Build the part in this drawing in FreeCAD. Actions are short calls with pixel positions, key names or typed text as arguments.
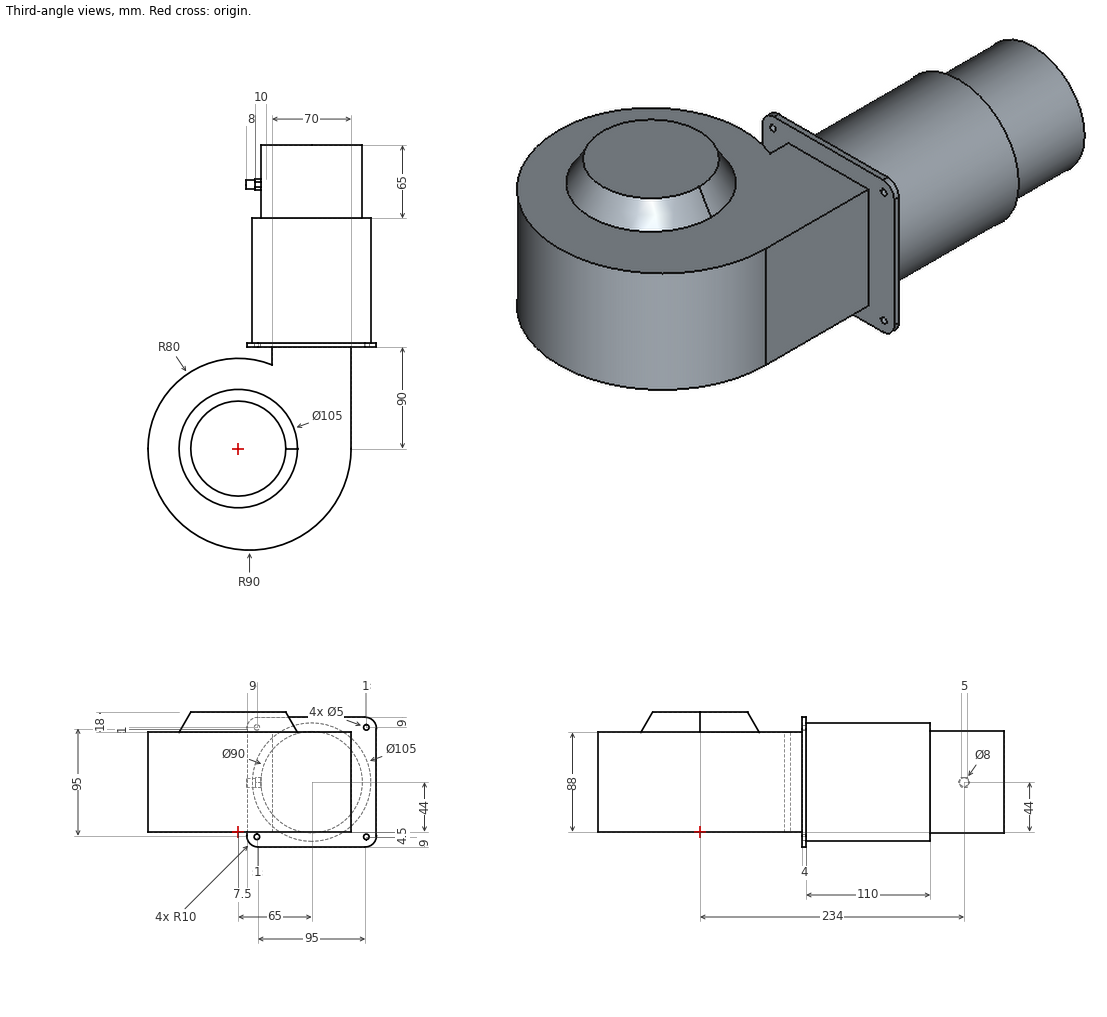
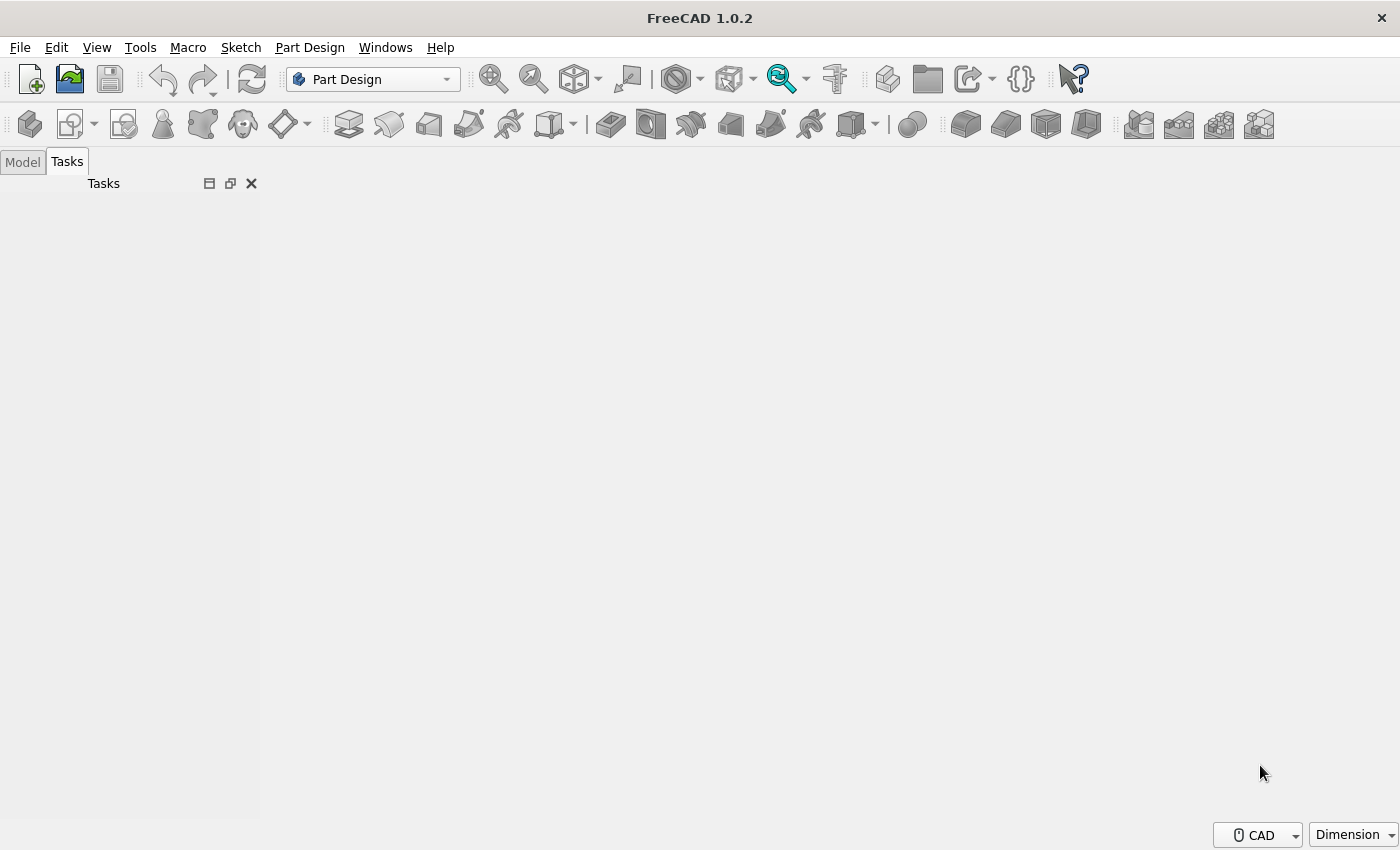
click(30, 80)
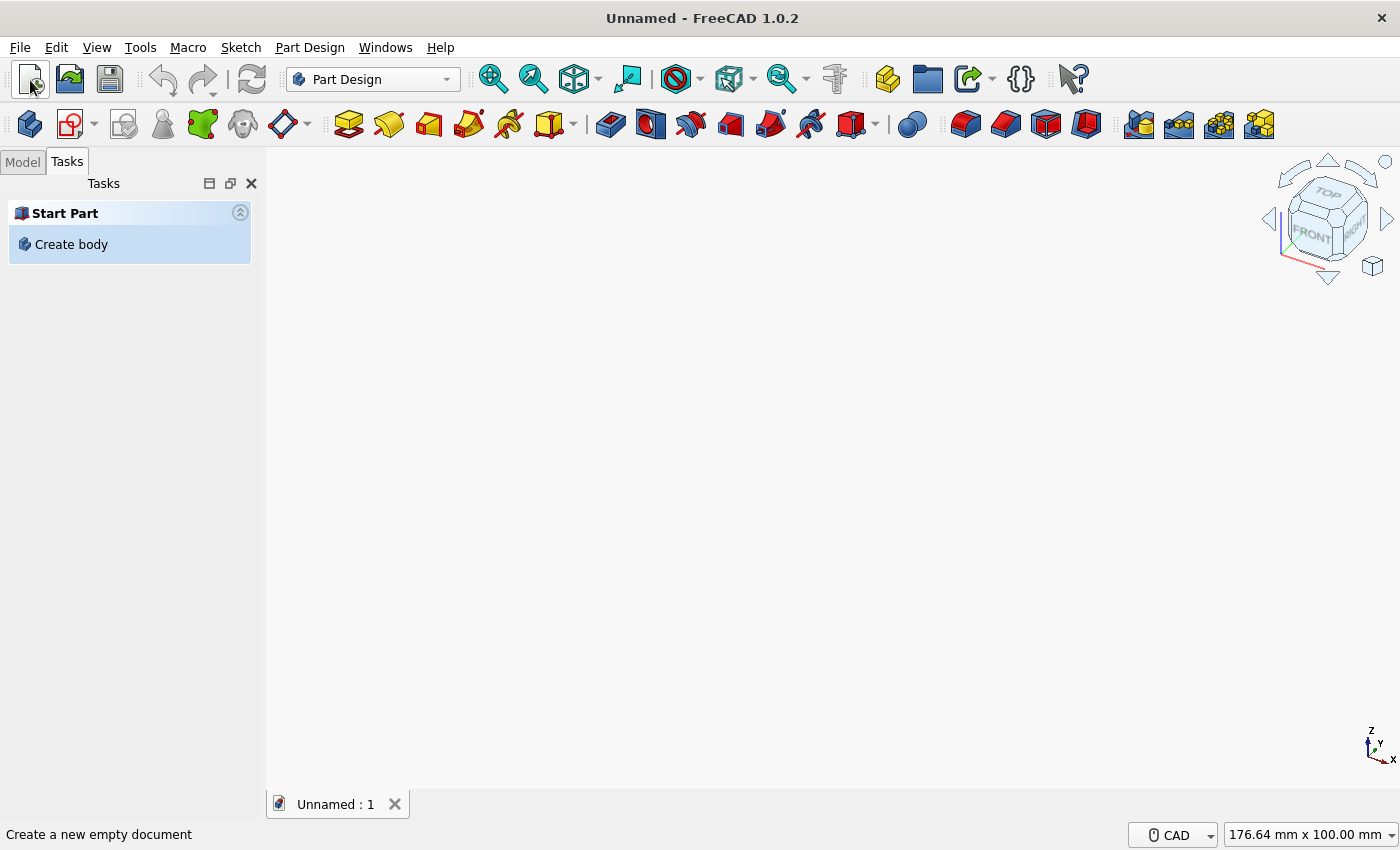
click(70, 124)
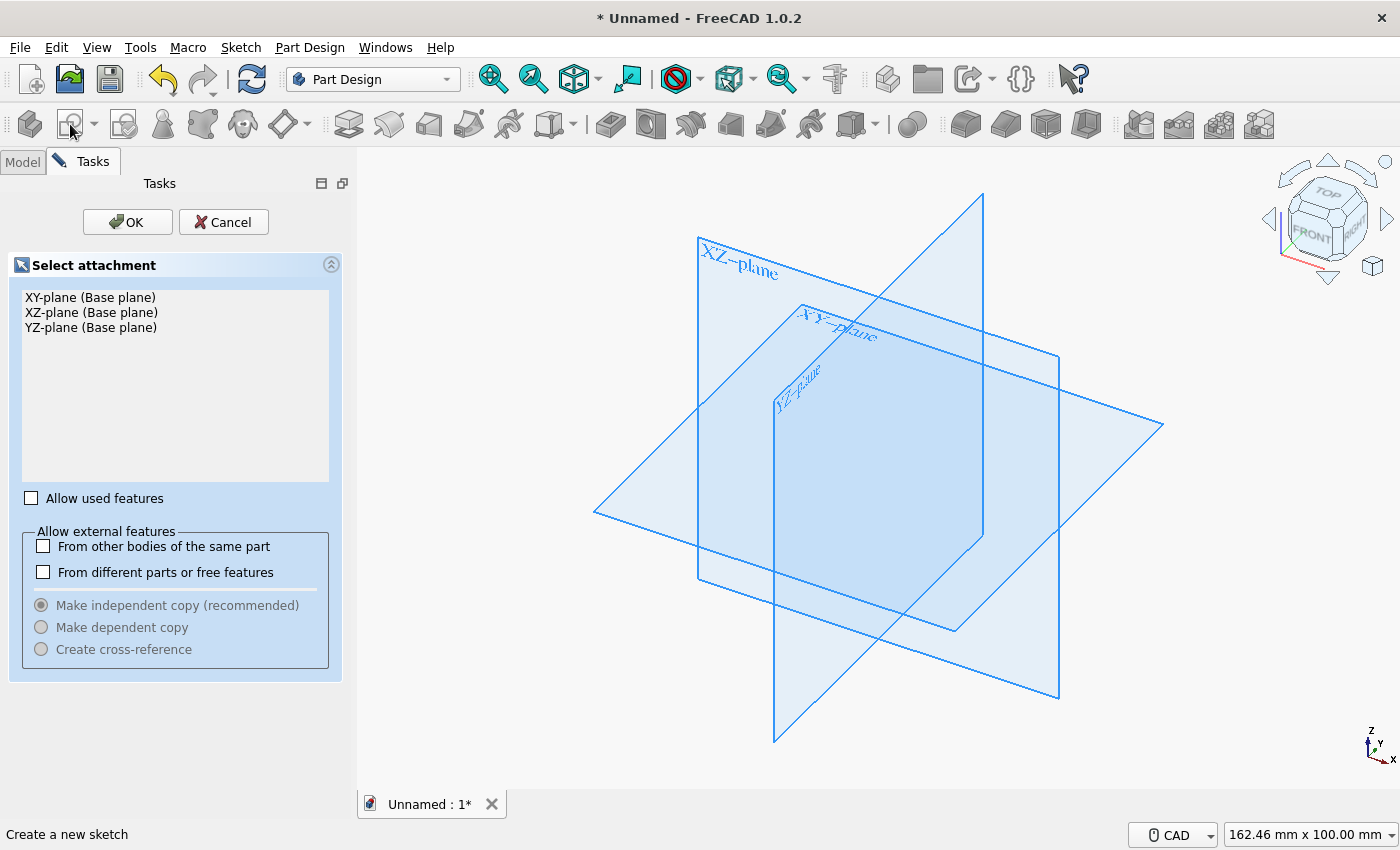
click(82, 298)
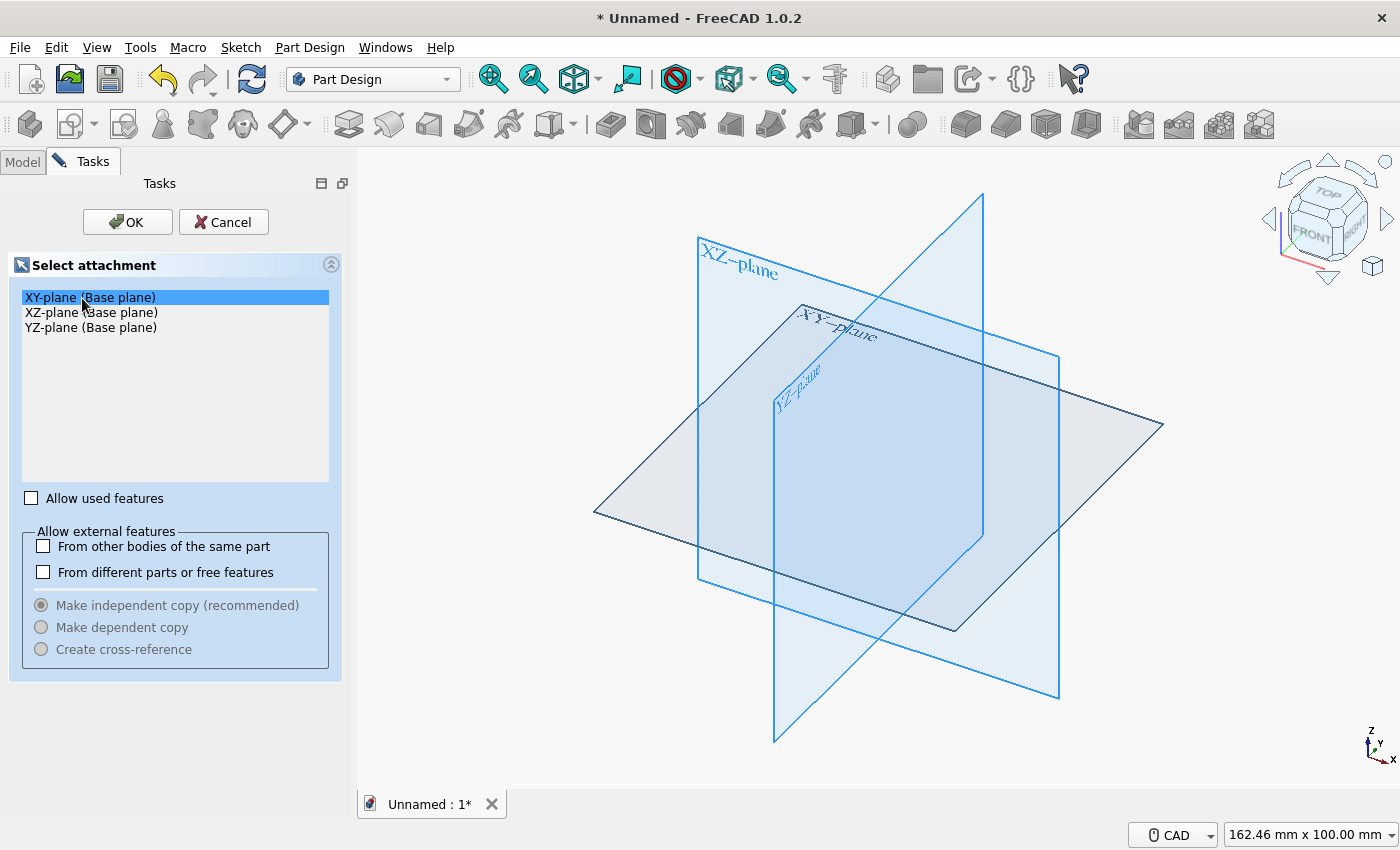
click(128, 222)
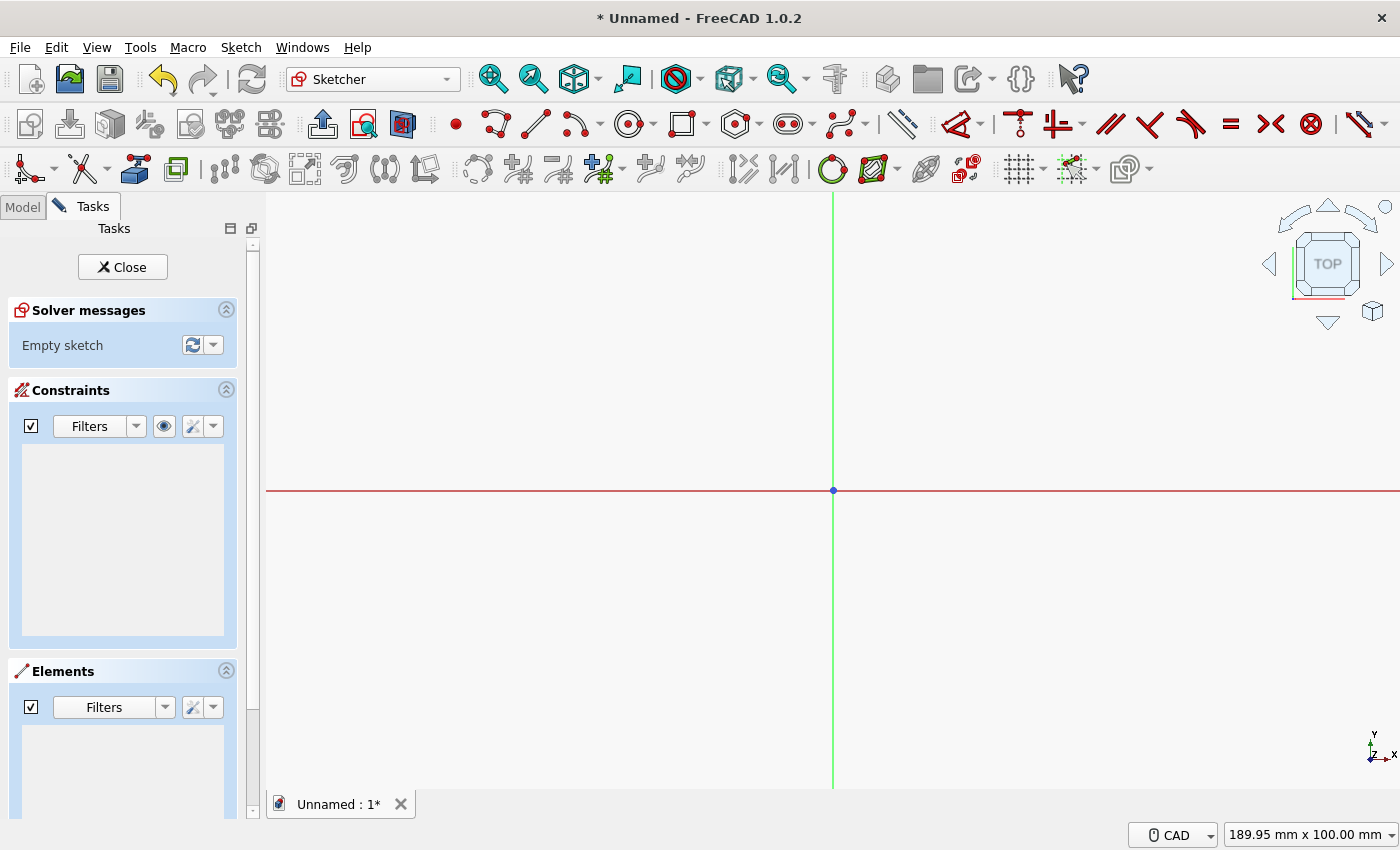
scroll(690, 490, down, 5)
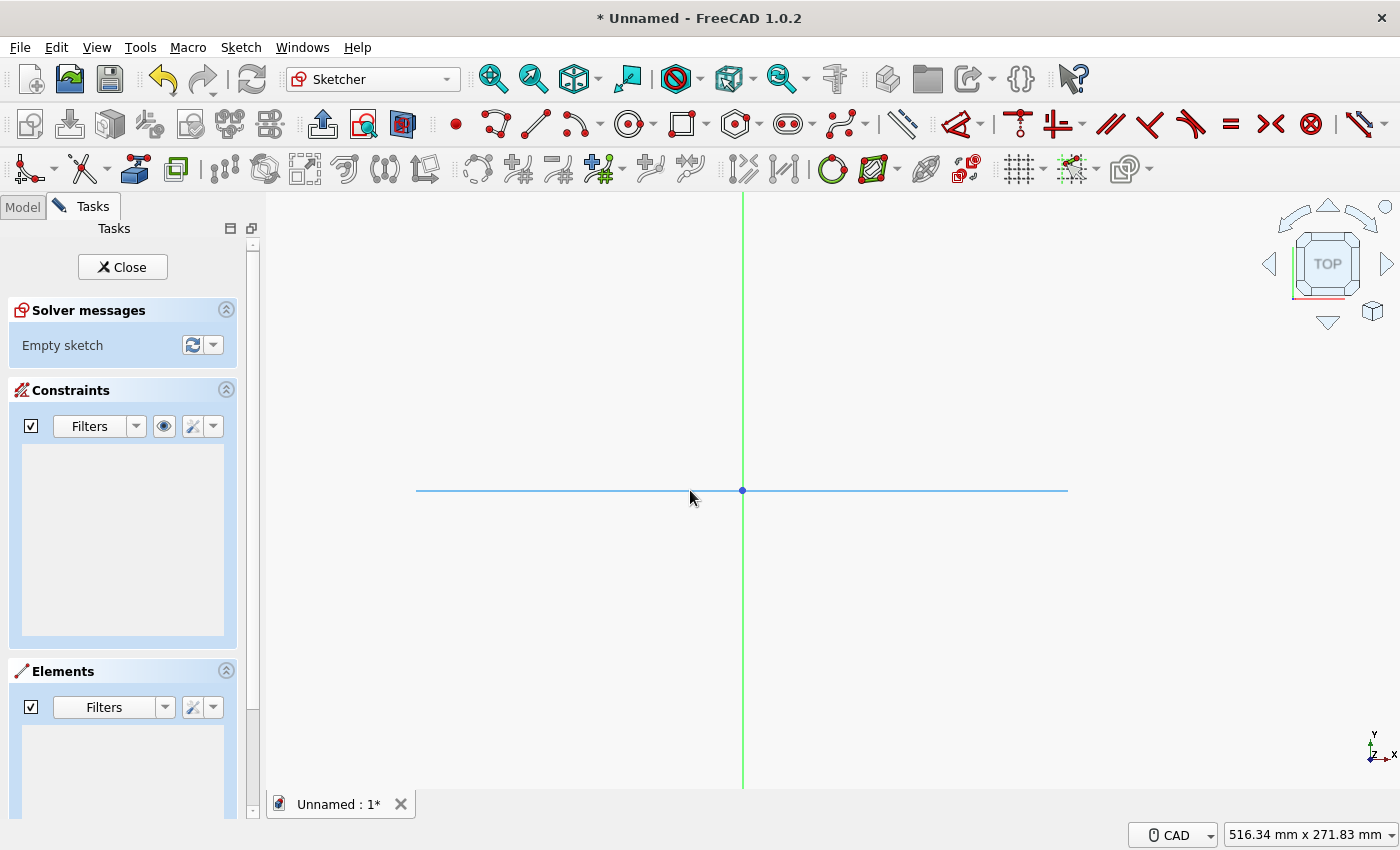
key(g)
key(m)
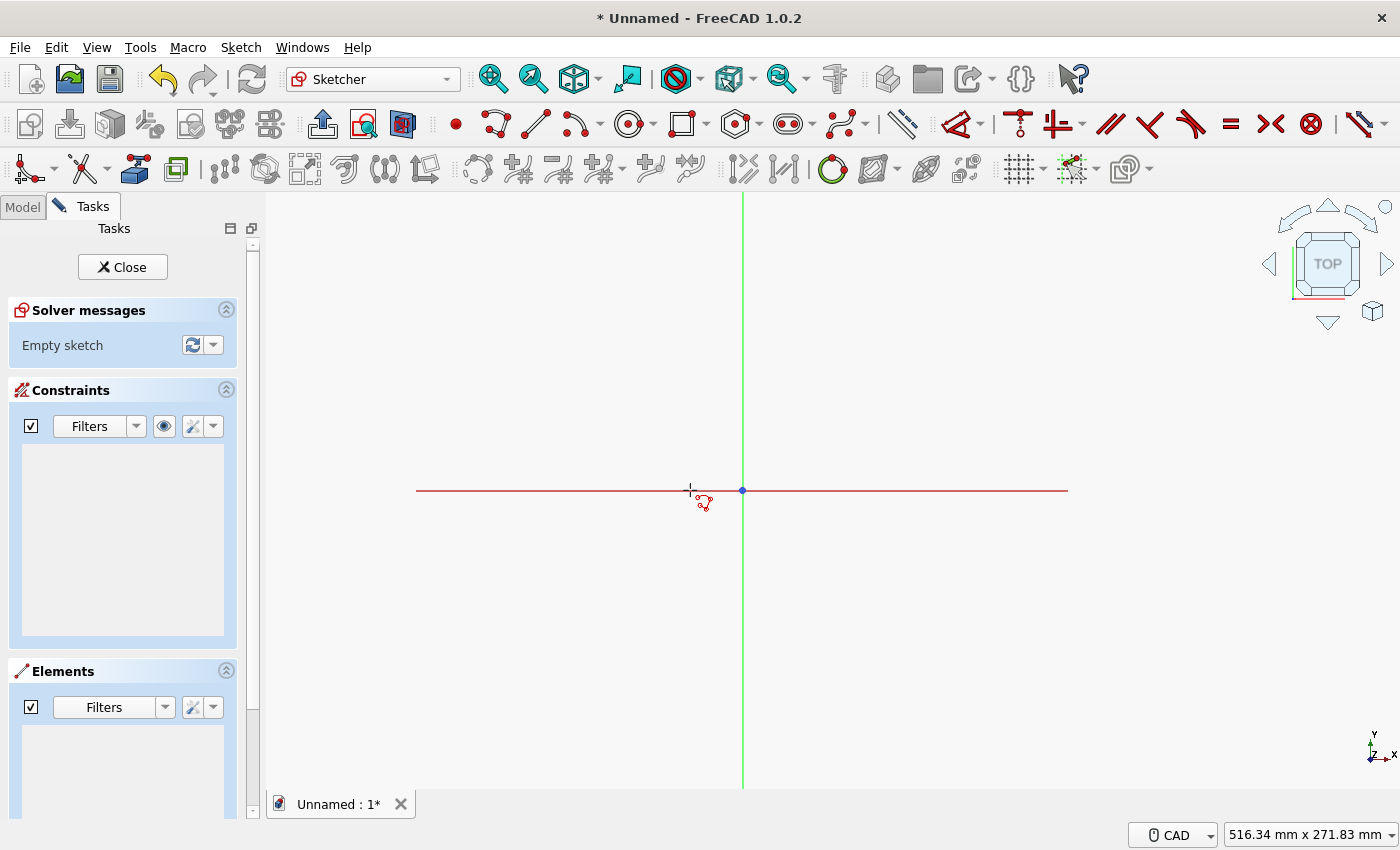
click(962, 490)
click(962, 293)
click(809, 293)
click(809, 328)
right_click(809, 328)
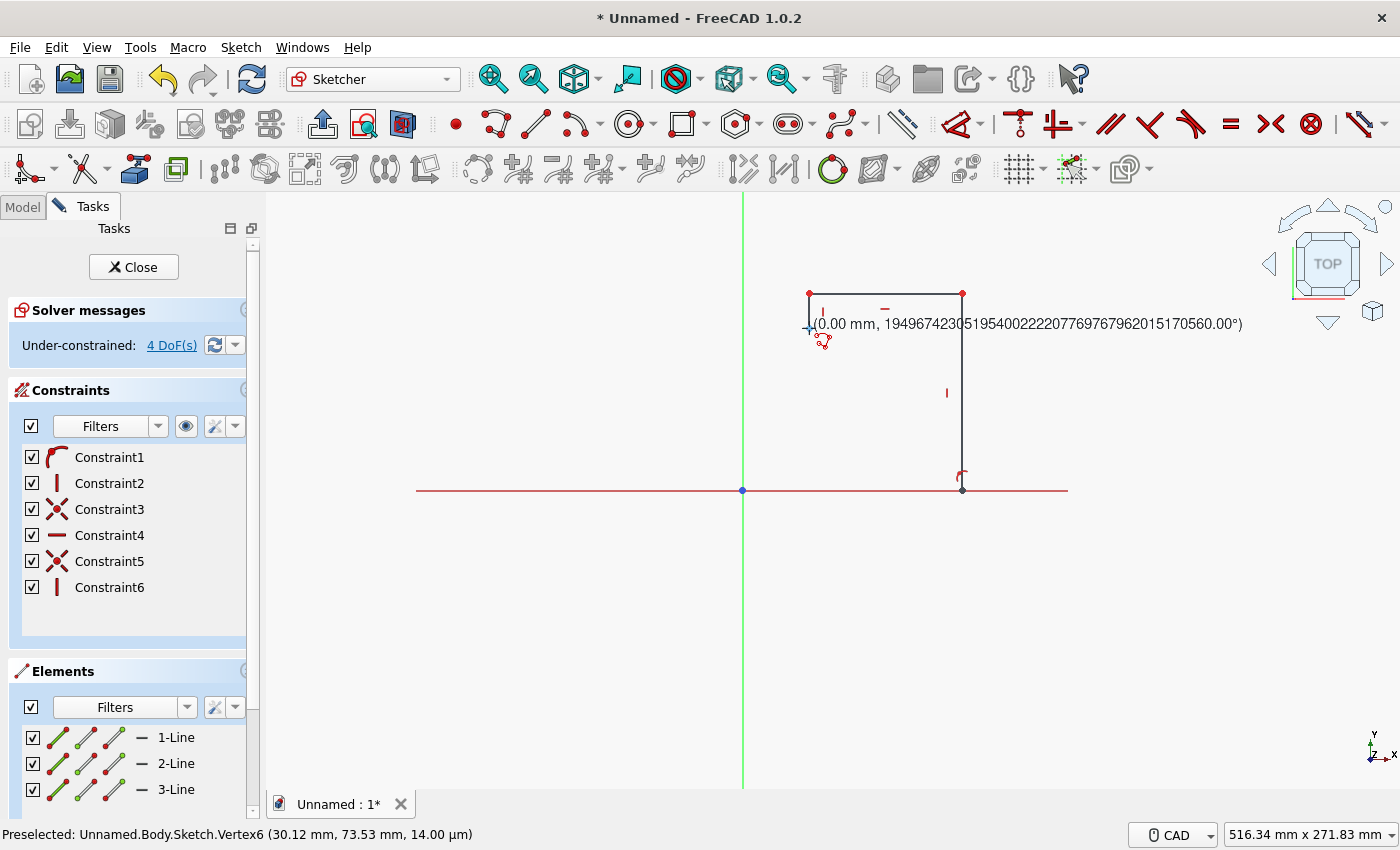
click(602, 124)